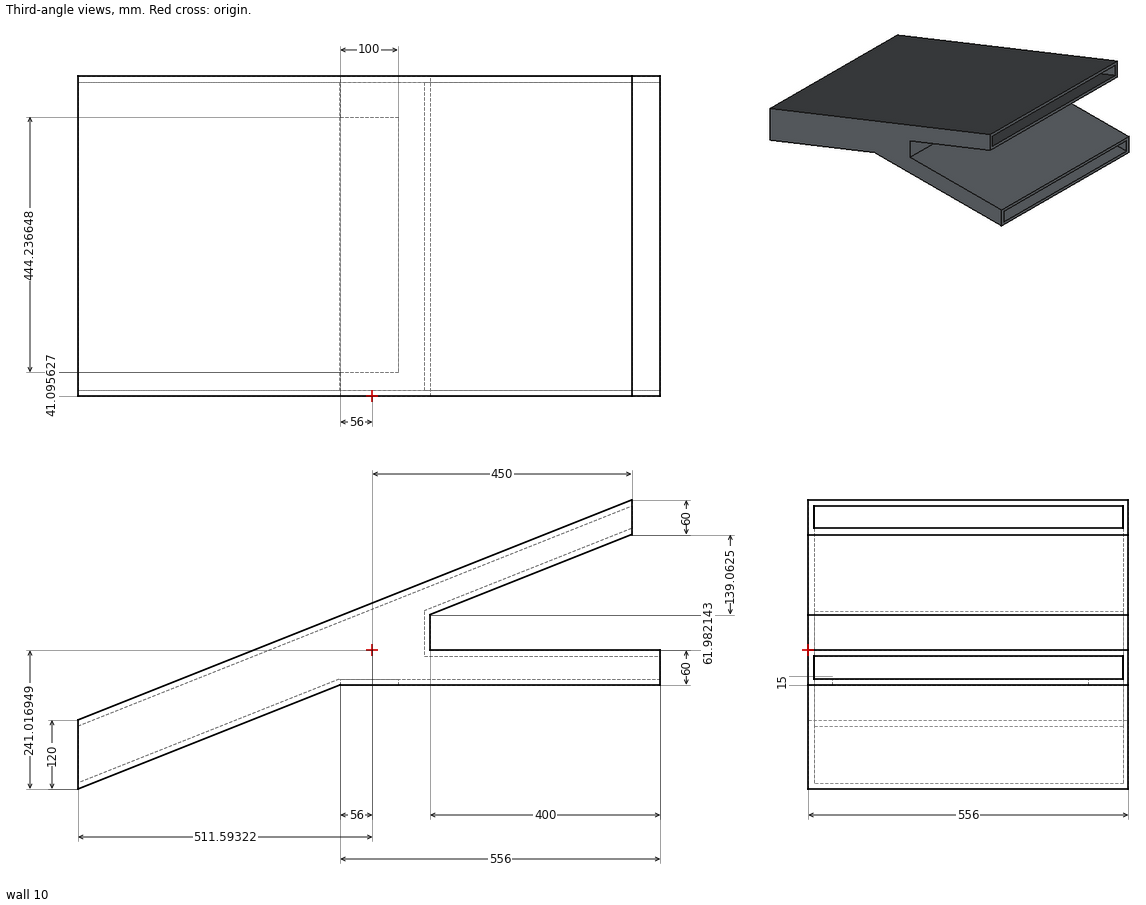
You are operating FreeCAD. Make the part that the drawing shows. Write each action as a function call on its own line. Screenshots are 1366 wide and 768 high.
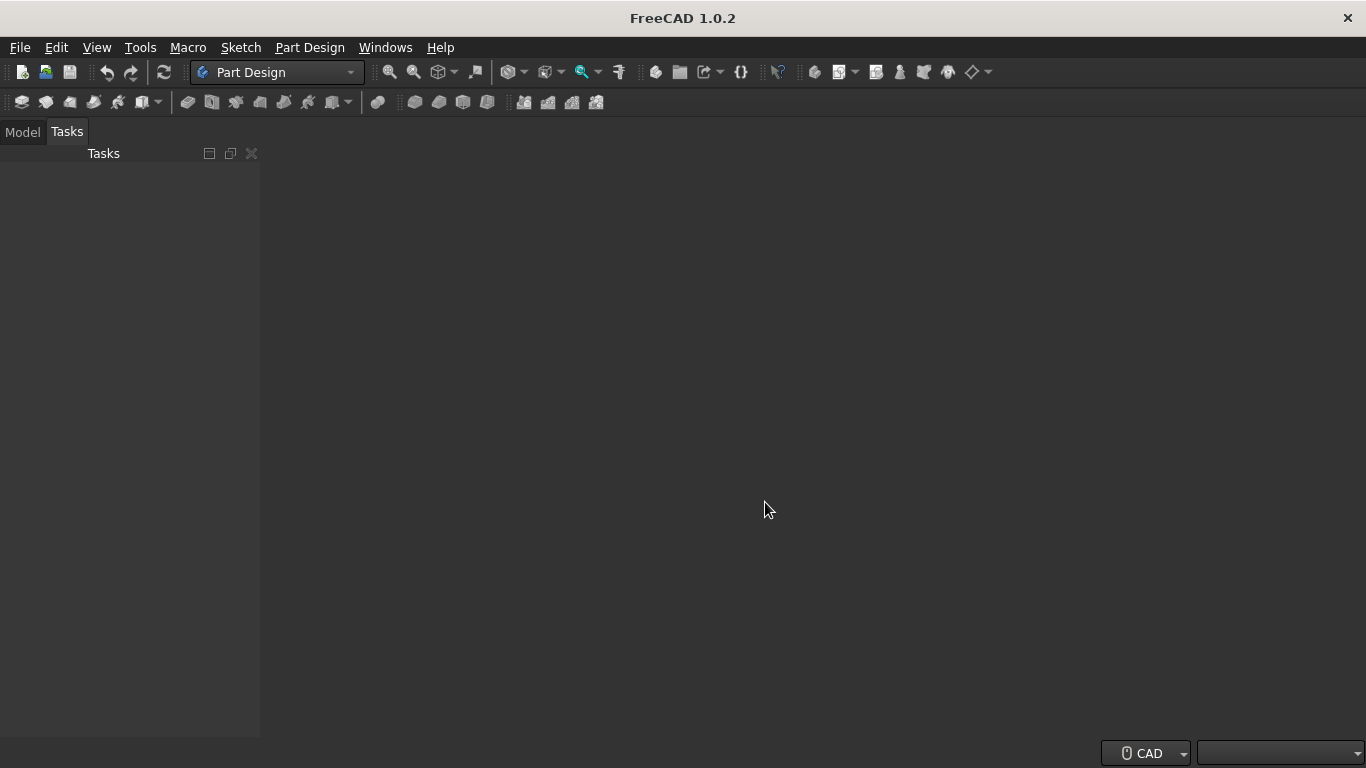
click(22, 72)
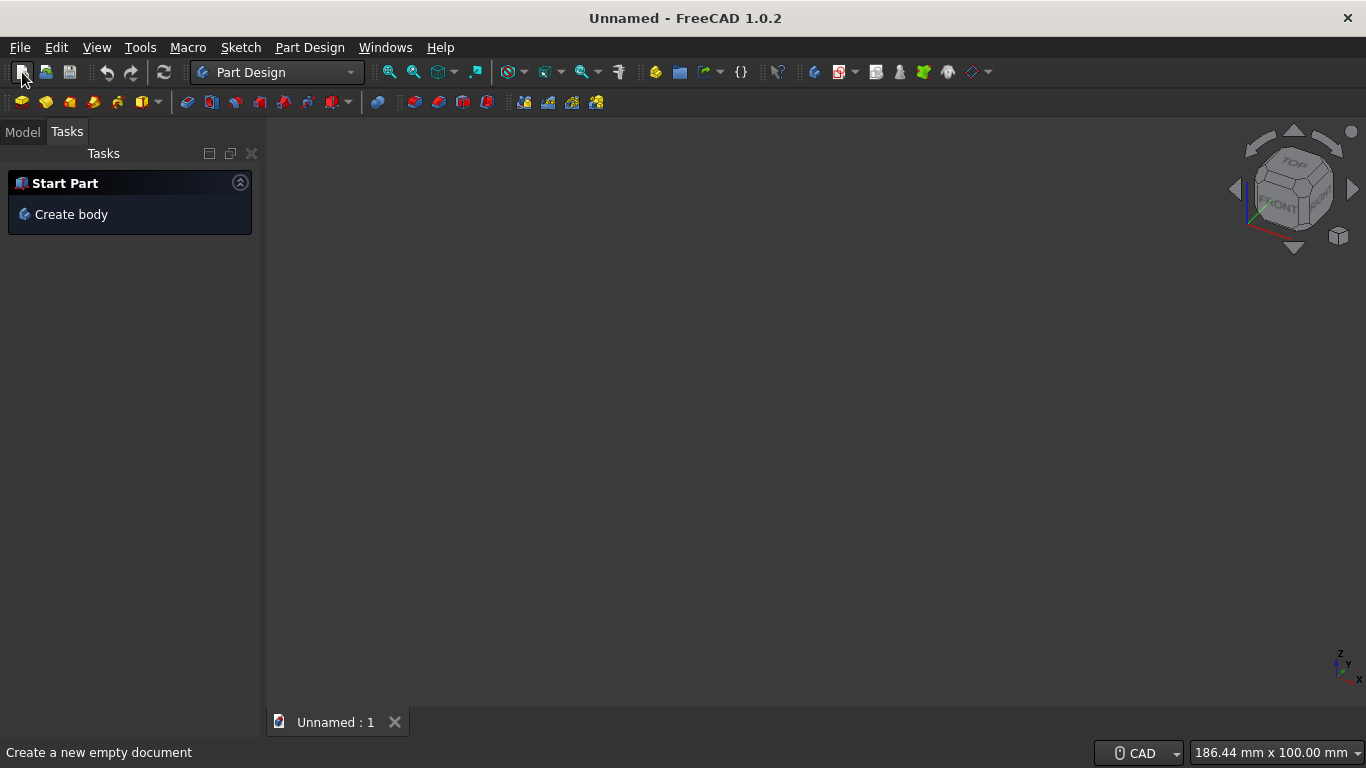
click(840, 72)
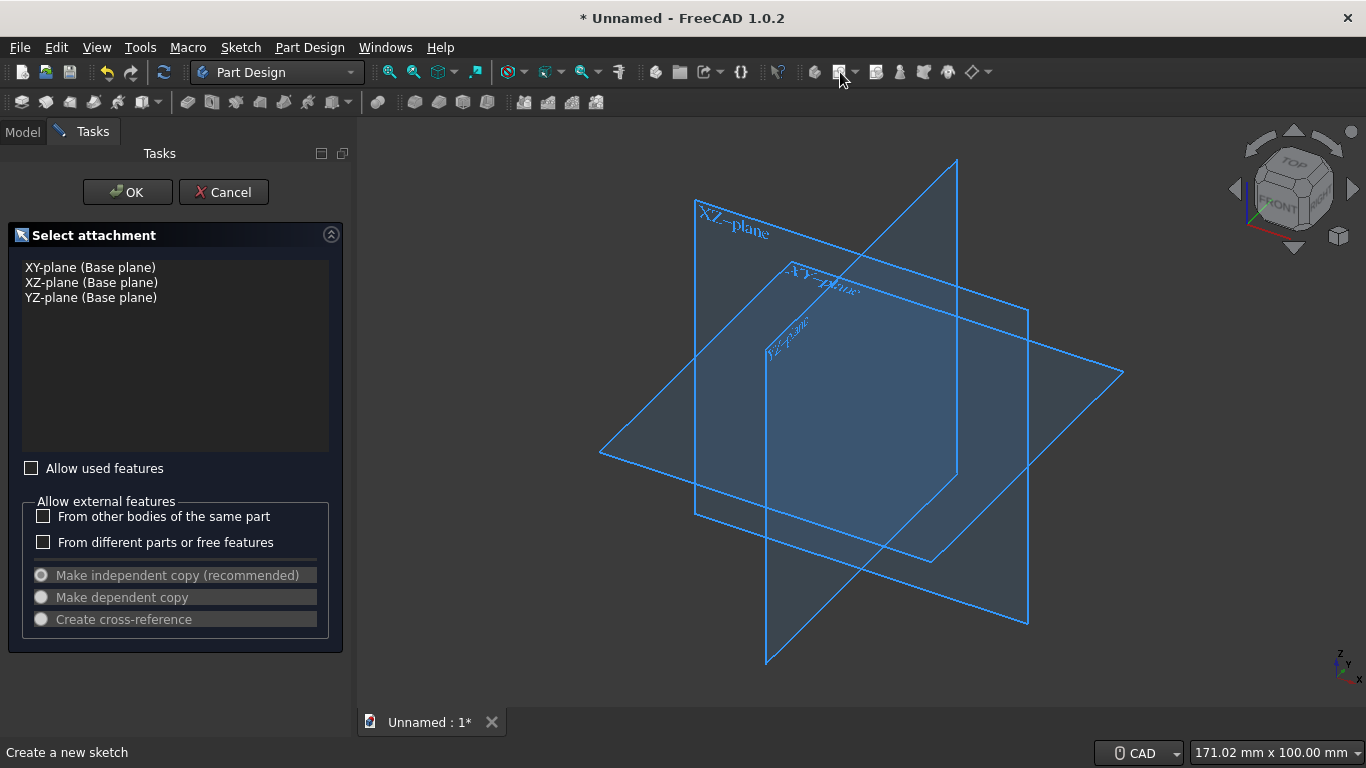
click(82, 282)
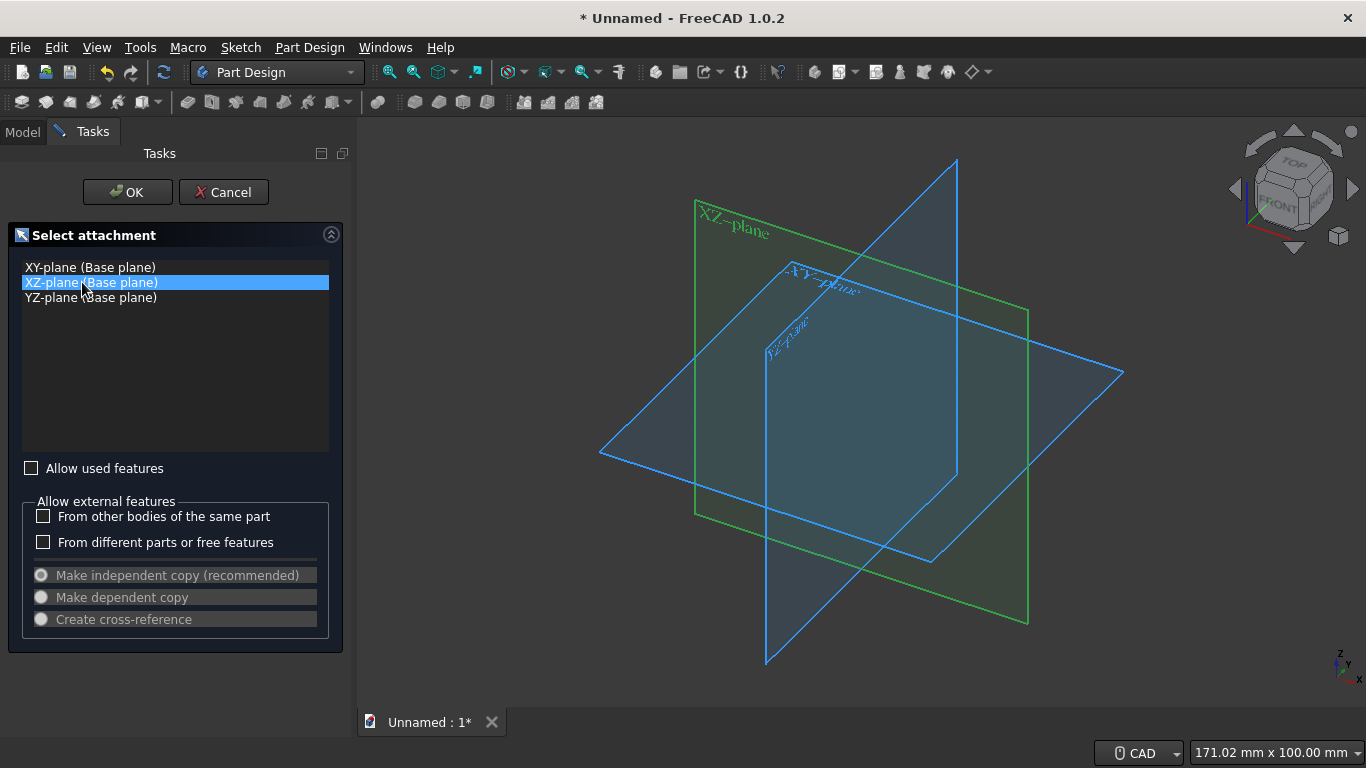
click(128, 192)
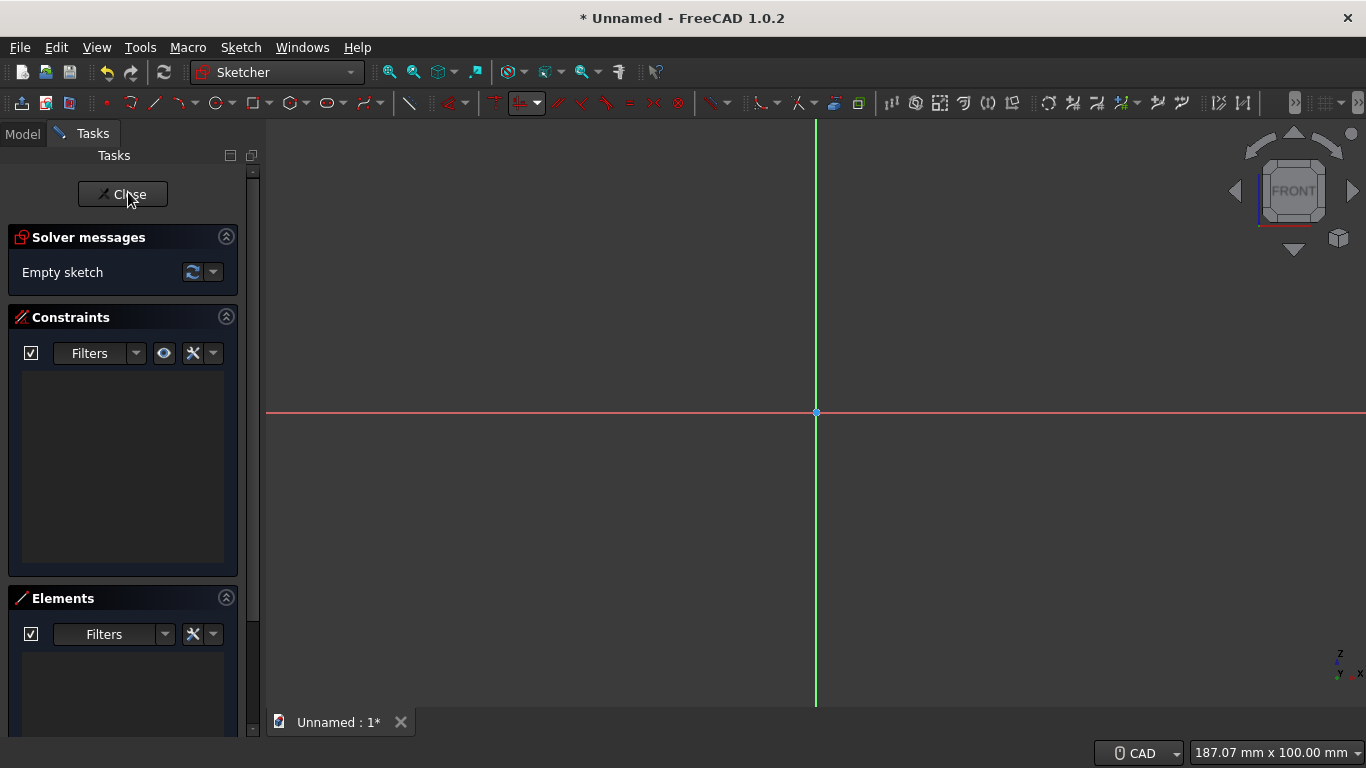
scroll(743, 420, down, 11)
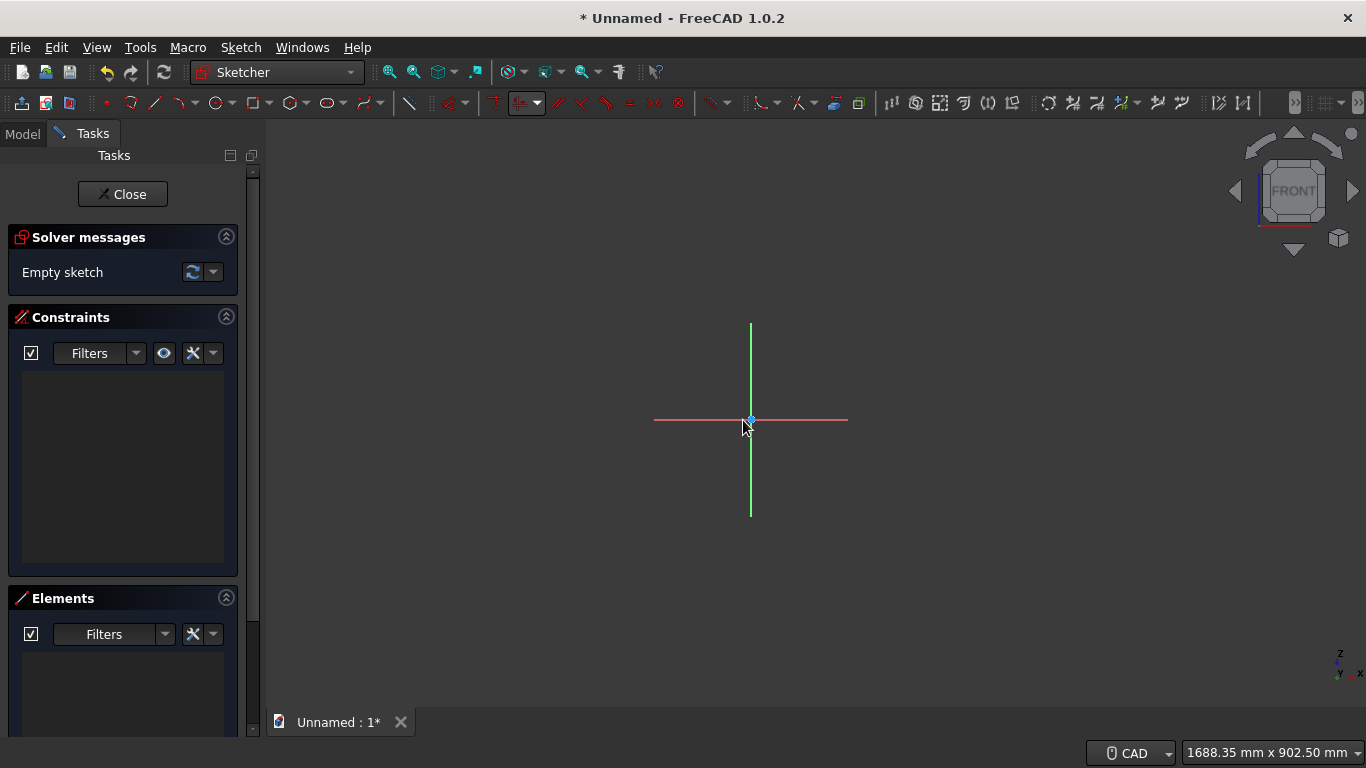
click(132, 104)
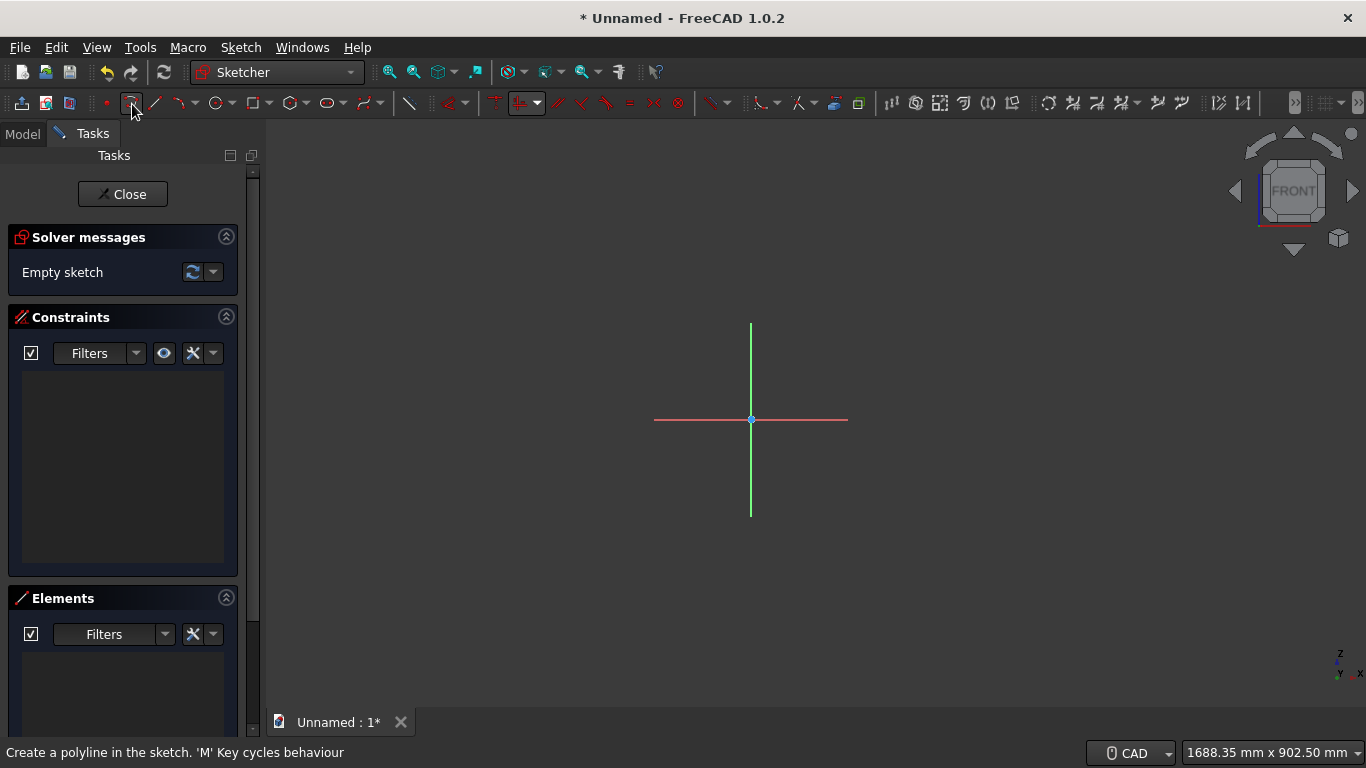
click(715, 459)
click(418, 577)
click(418, 499)
click(1045, 250)
click(1045, 289)
click(817, 379)
click(817, 420)
click(1077, 411)
click(1077, 459)
click(715, 460)
key(Escape)
key(Escape)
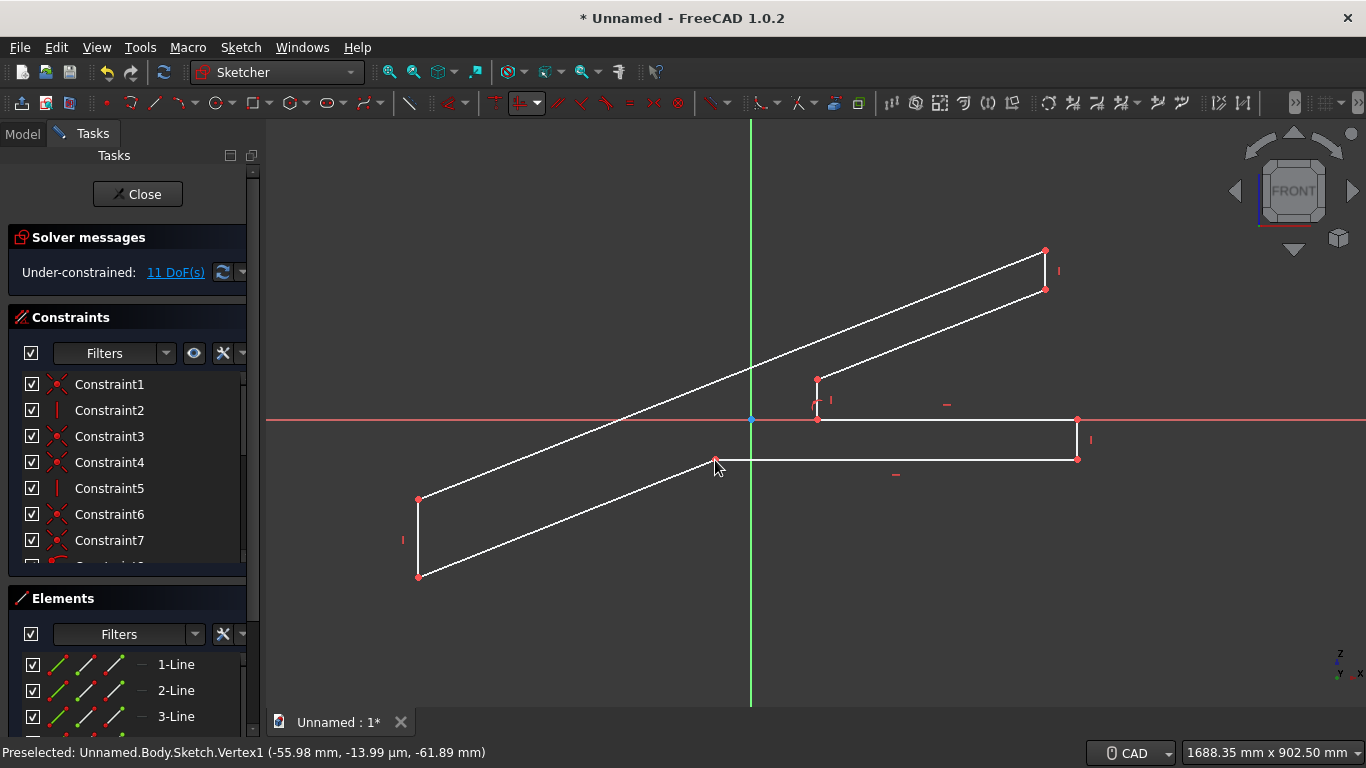
click(448, 104)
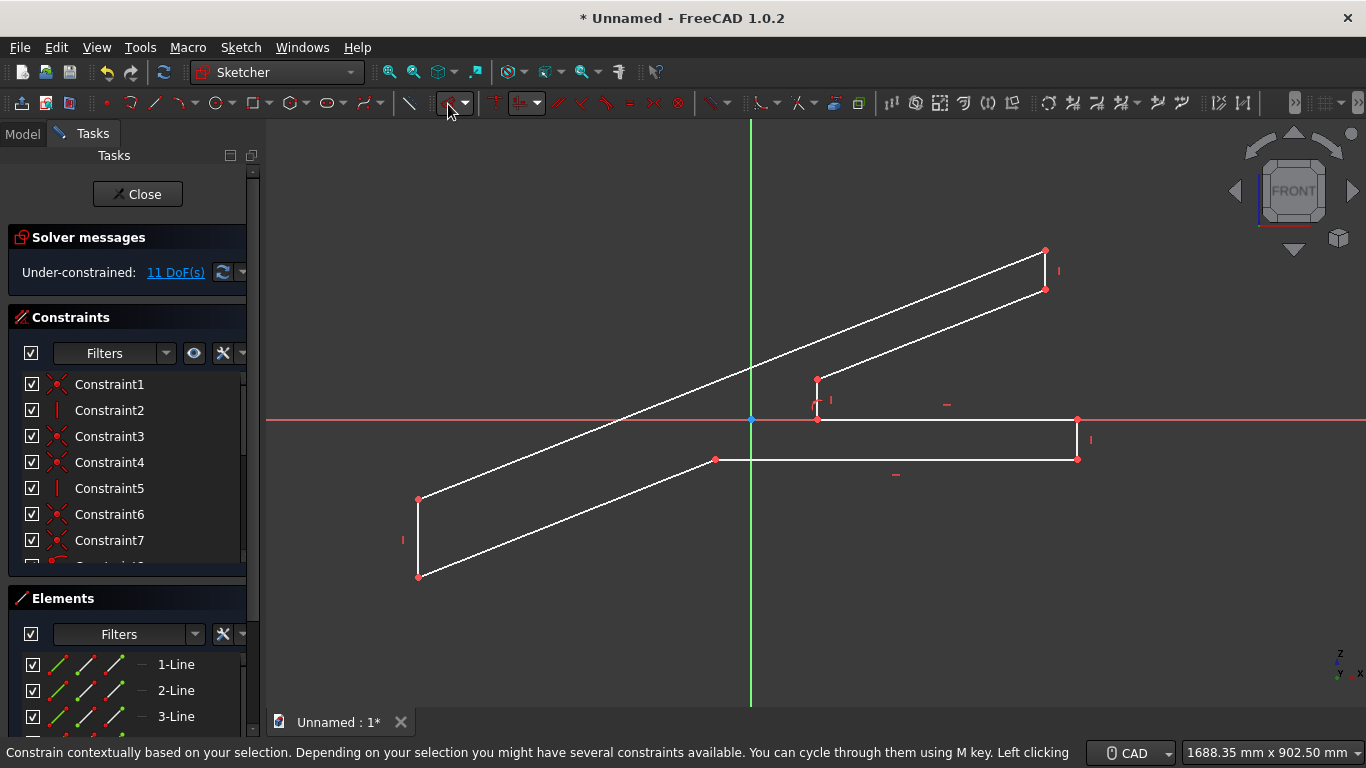
scroll(1045, 263, up, 2)